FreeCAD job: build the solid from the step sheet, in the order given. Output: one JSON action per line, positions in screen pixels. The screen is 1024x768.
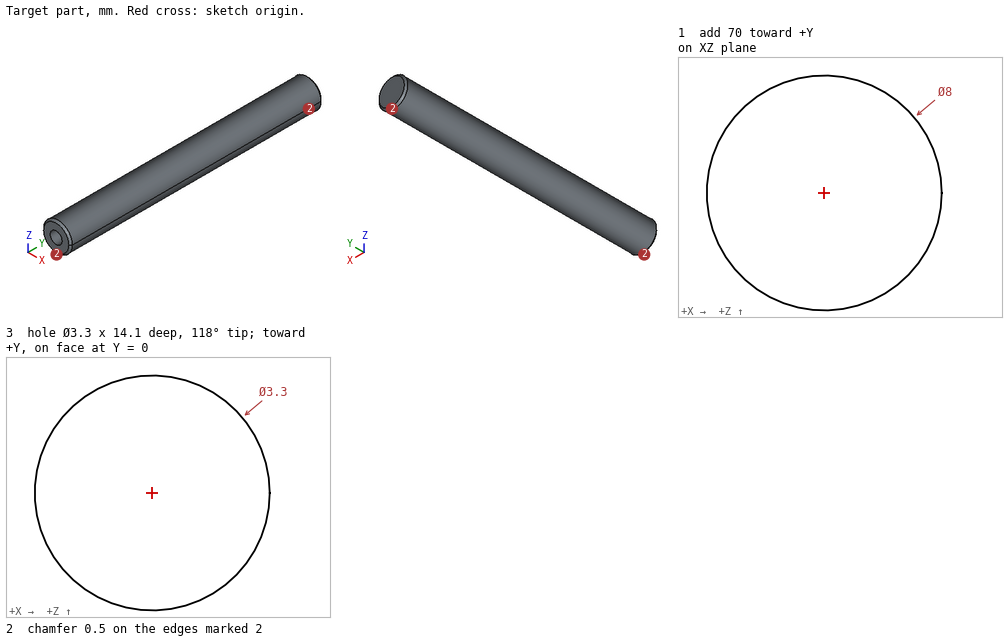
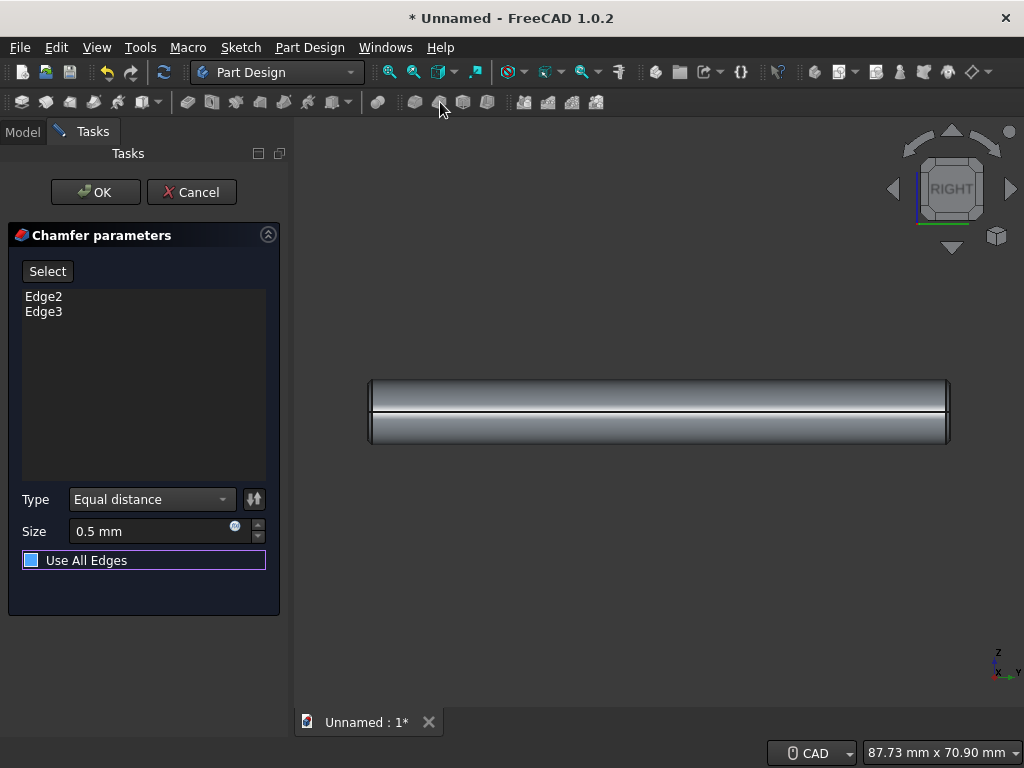
{"action": "left_click", "coordinate": [96, 192]}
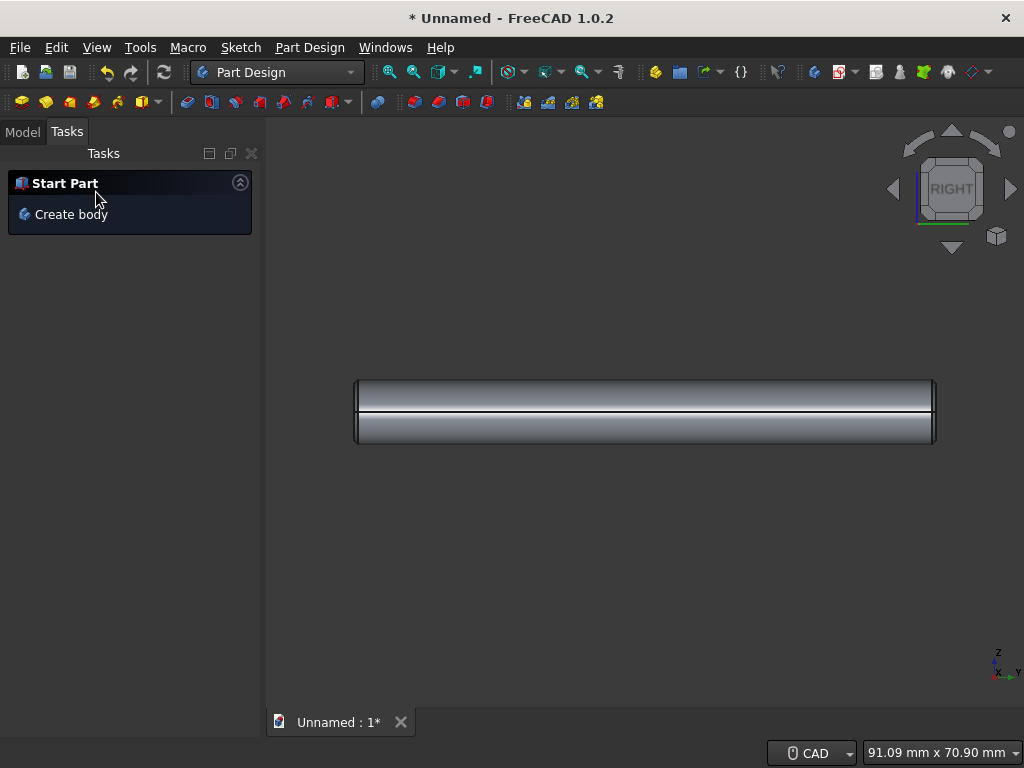
{"action": "key", "text": "0"}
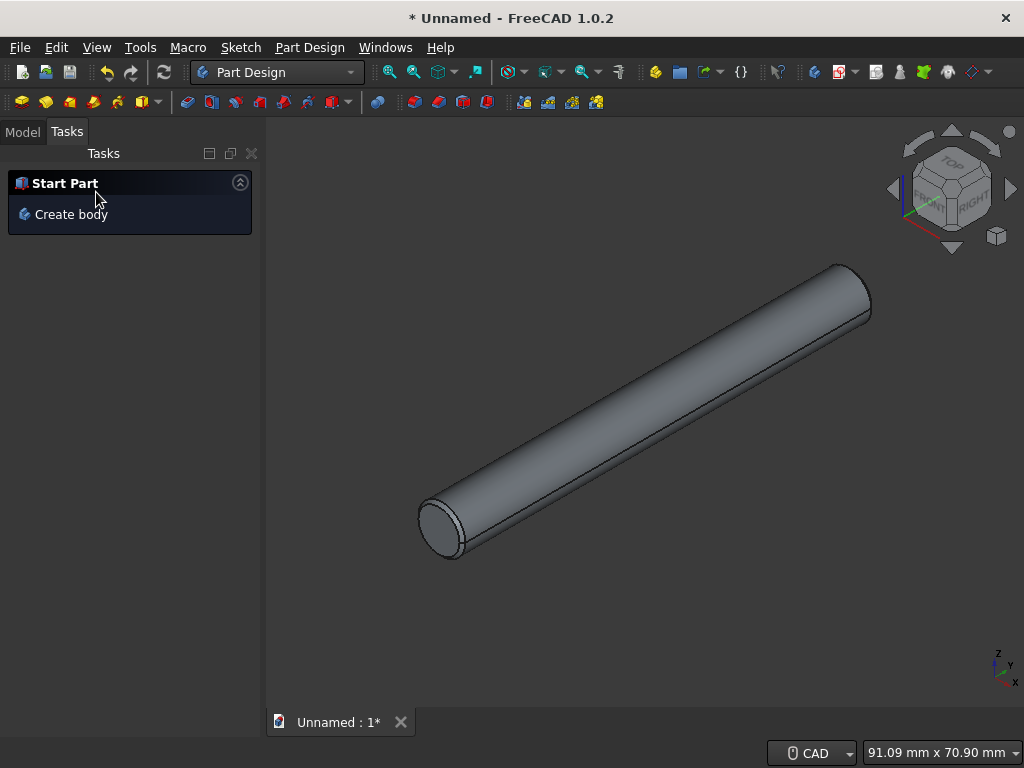
{"action": "left_click", "coordinate": [439, 530]}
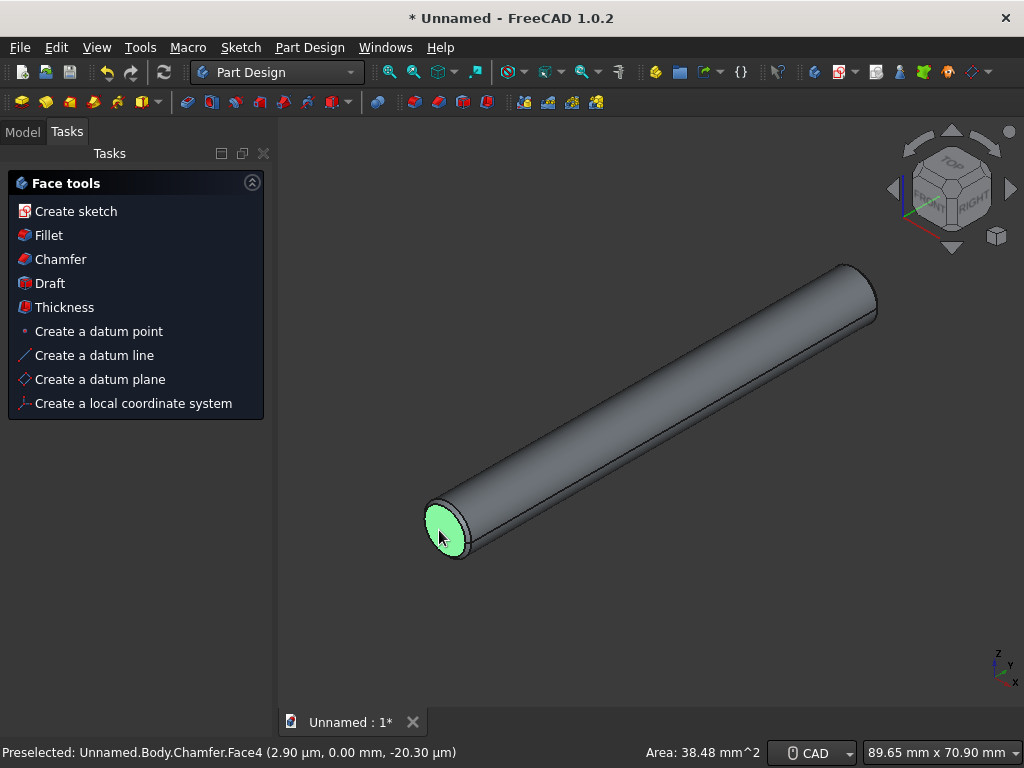
{"action": "left_click", "coordinate": [840, 72]}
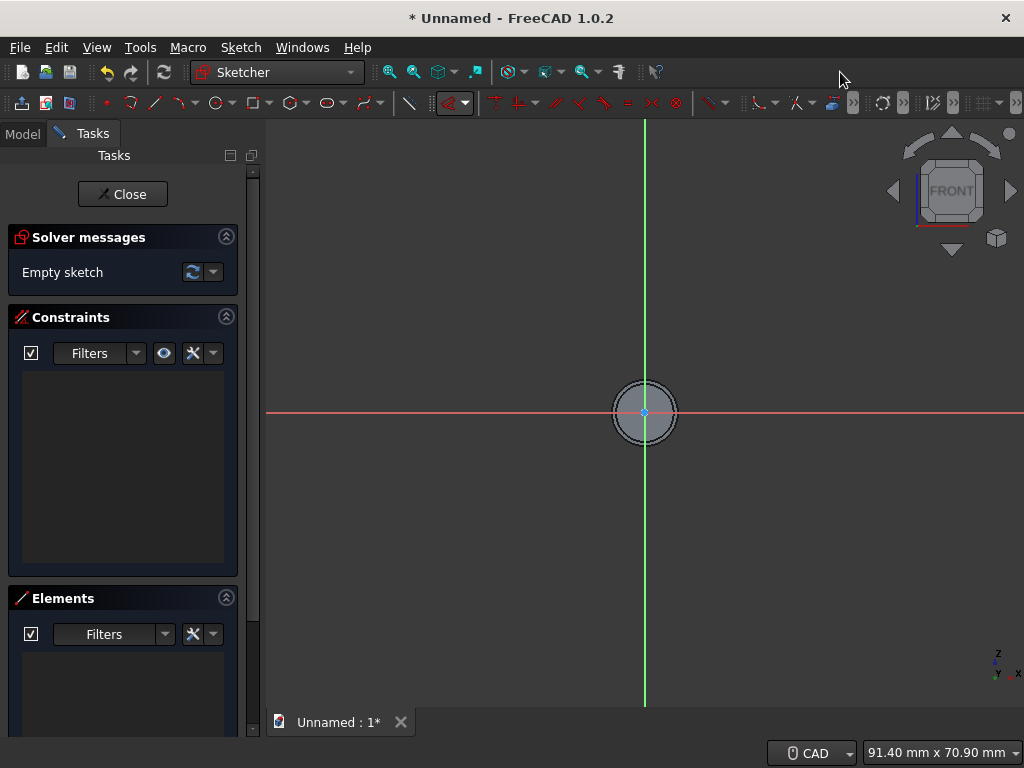
{"action": "scroll", "coordinate": [650, 413], "scroll_direction": "up", "scroll_amount": 13}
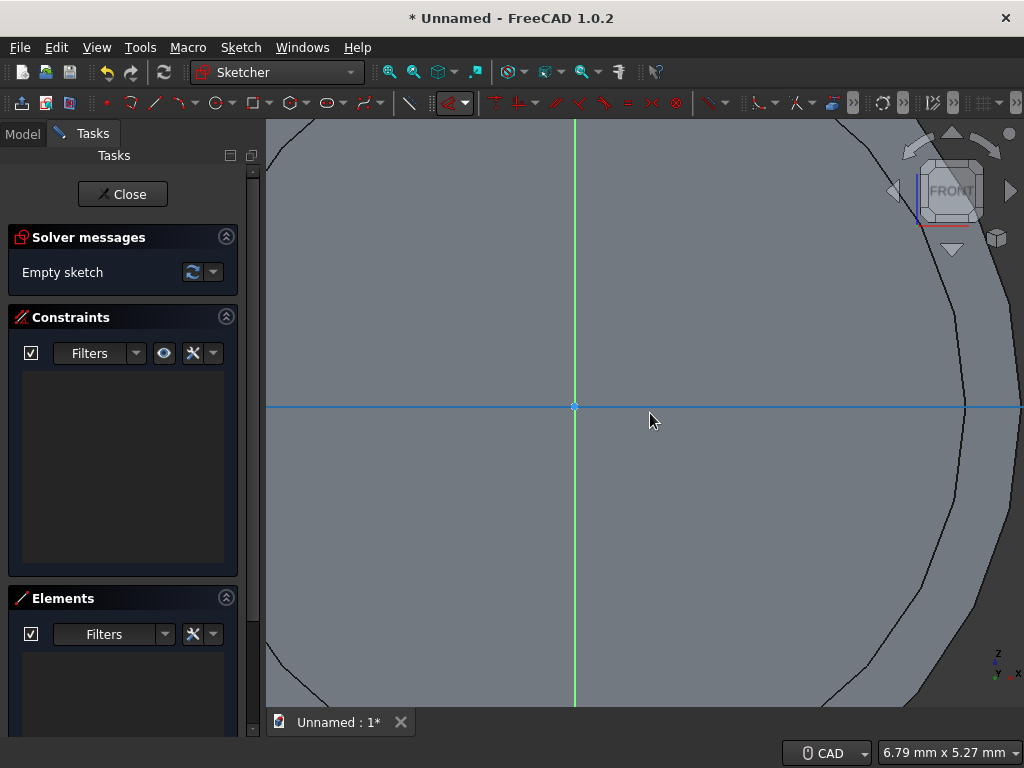
{"action": "key", "text": "g c"}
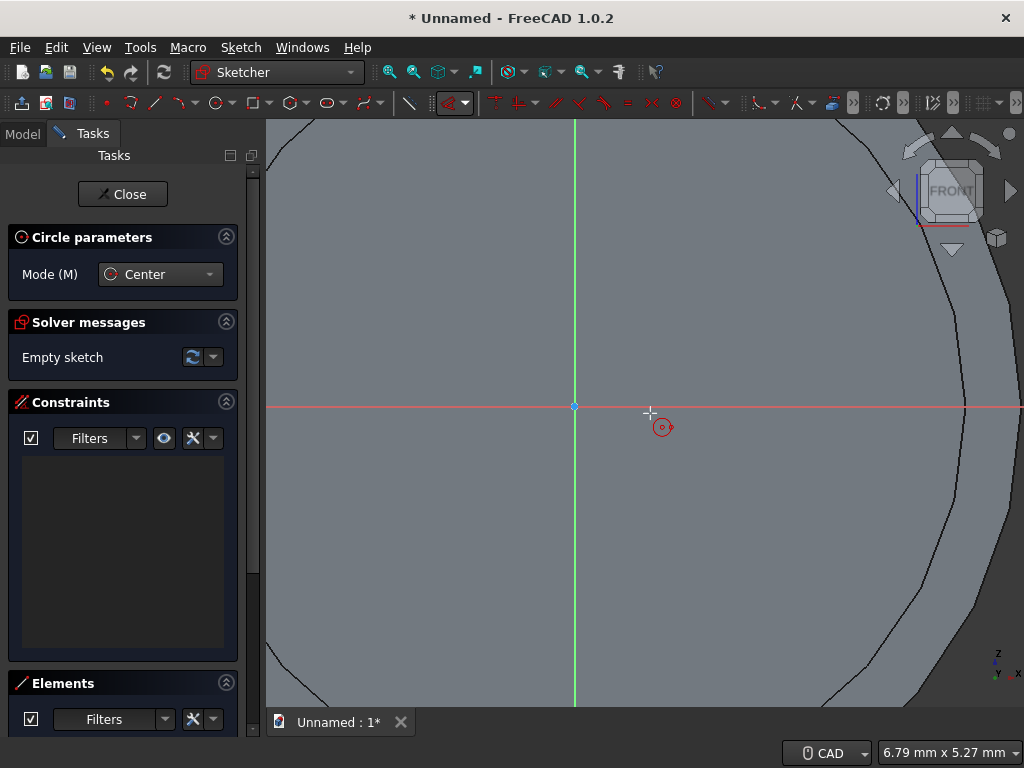
{"action": "left_click", "coordinate": [575, 407]}
{"action": "left_click", "coordinate": [705, 276]}
{"action": "key", "text": "Escape"}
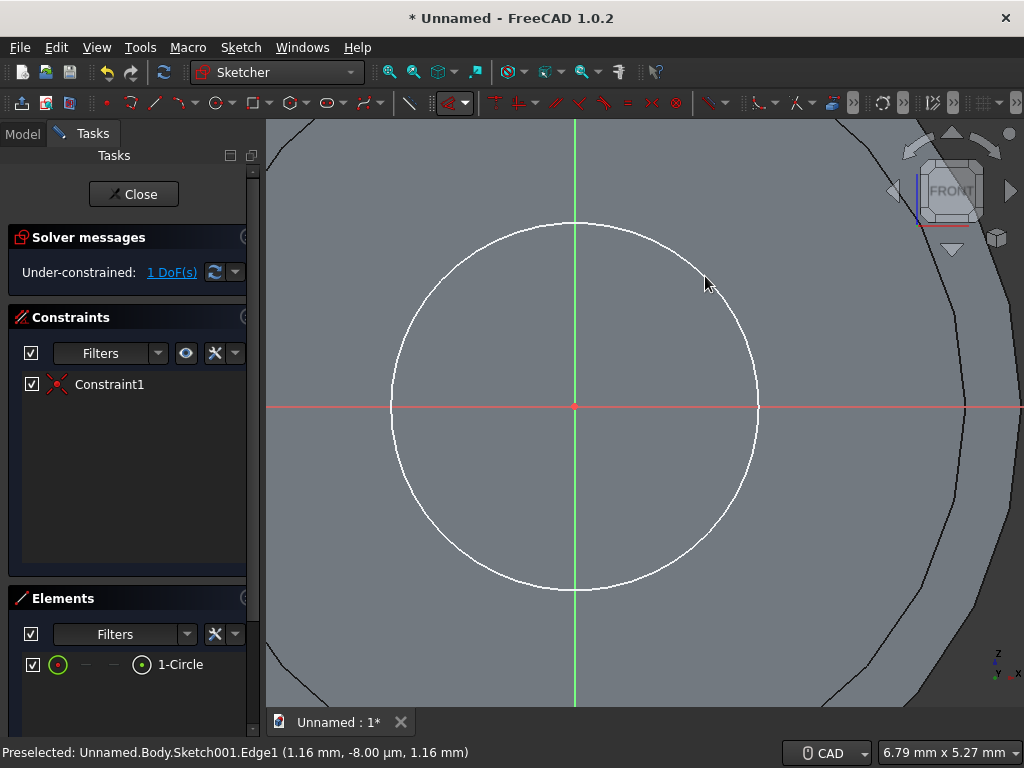
{"action": "left_click", "coordinate": [704, 276]}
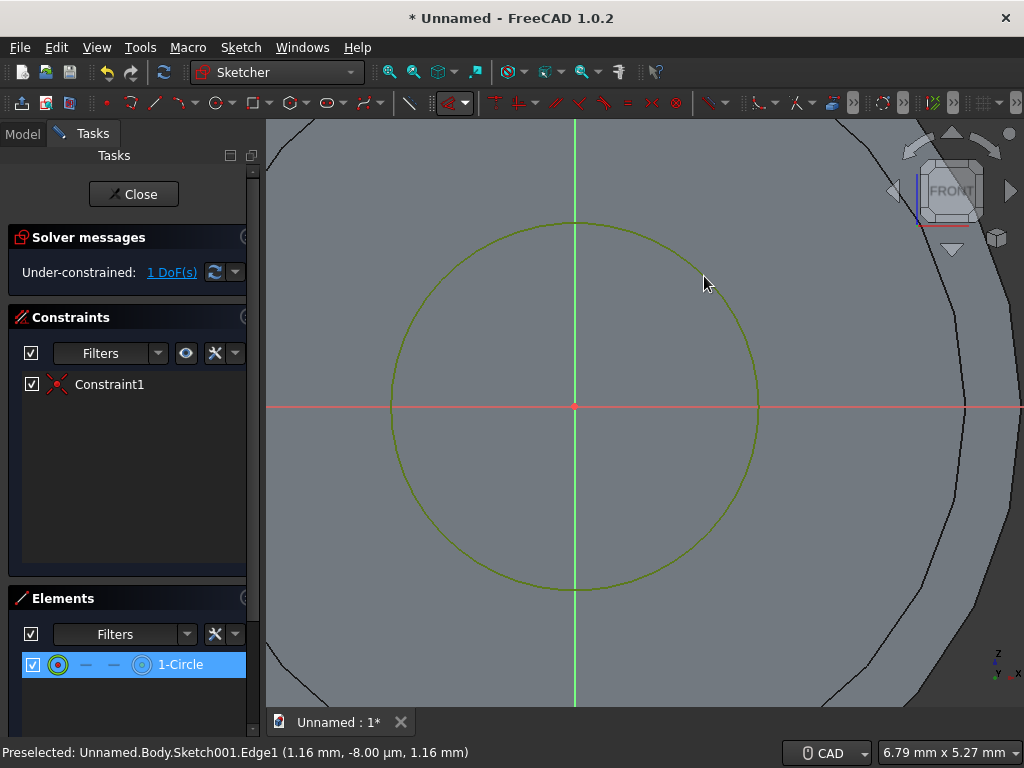
{"action": "key", "text": "k o"}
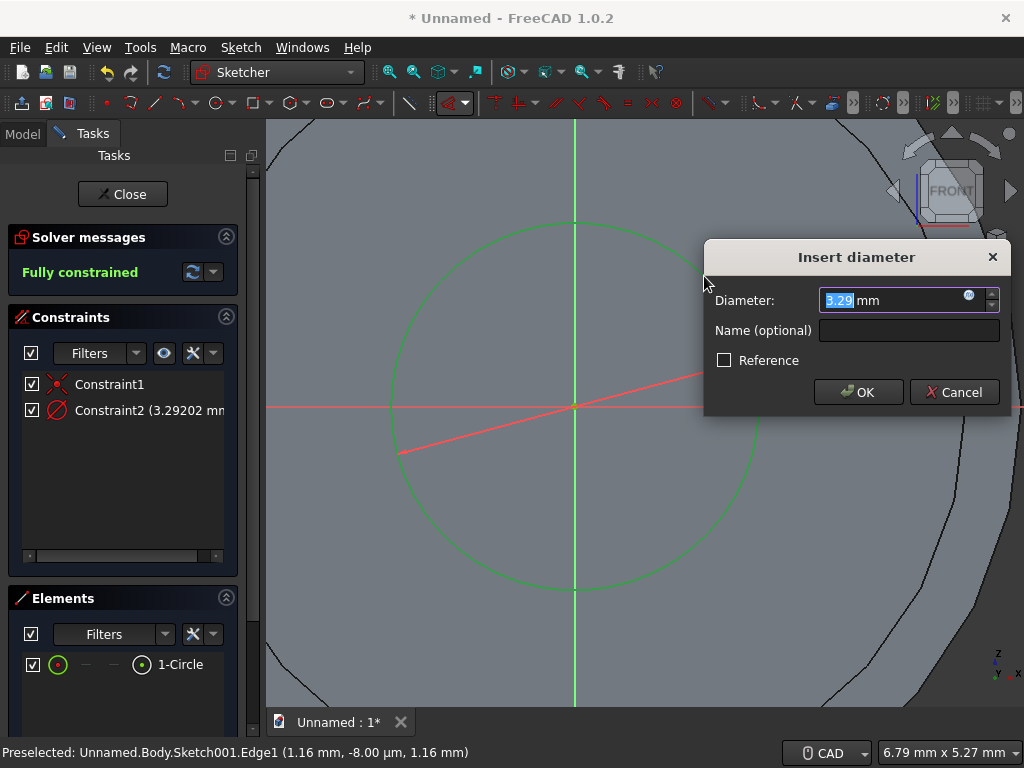
{"action": "type", "text": "3.3"}
{"action": "key", "text": "Return"}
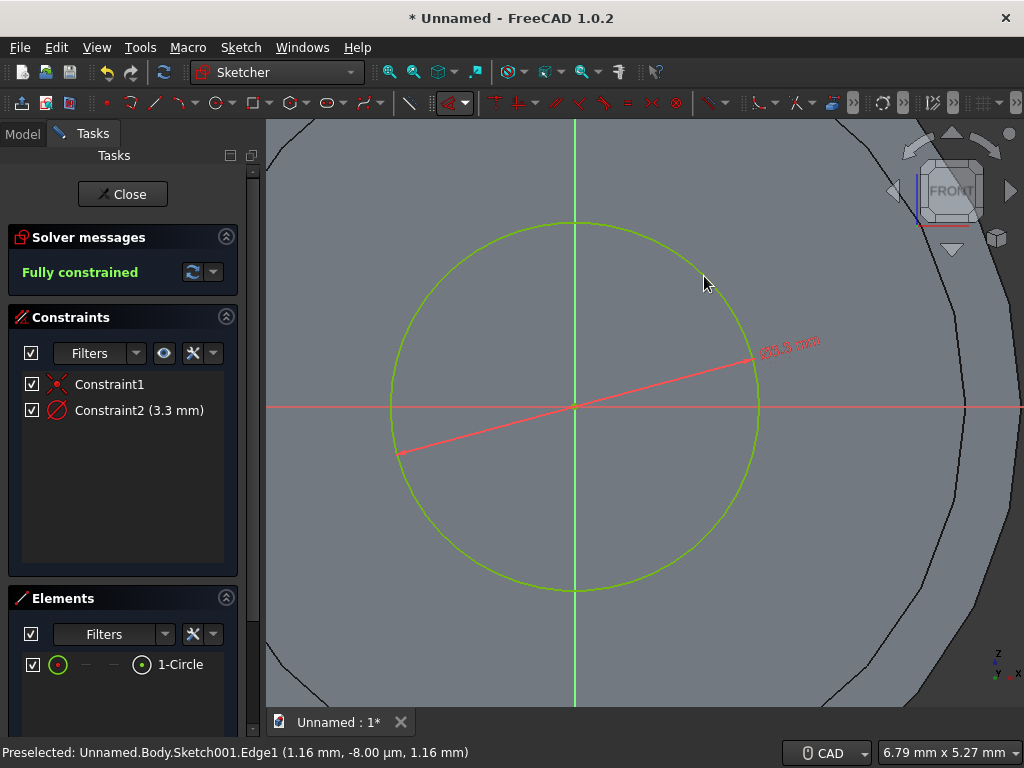
{"action": "left_click", "coordinate": [123, 194]}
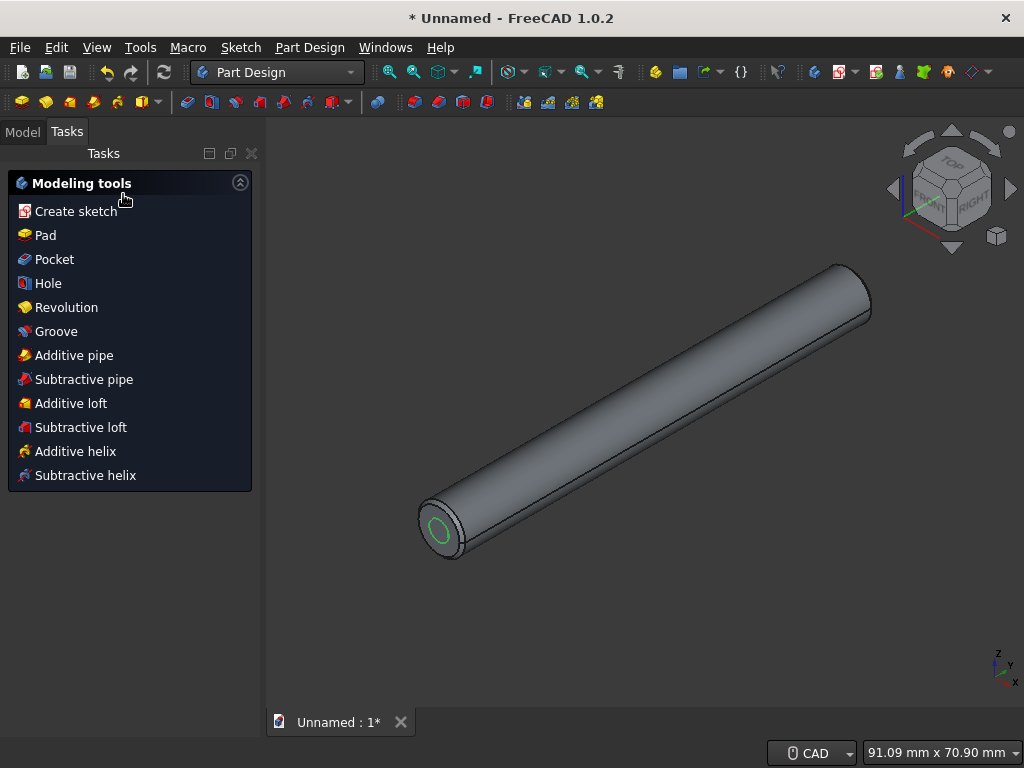
{"action": "left_click", "coordinate": [212, 102]}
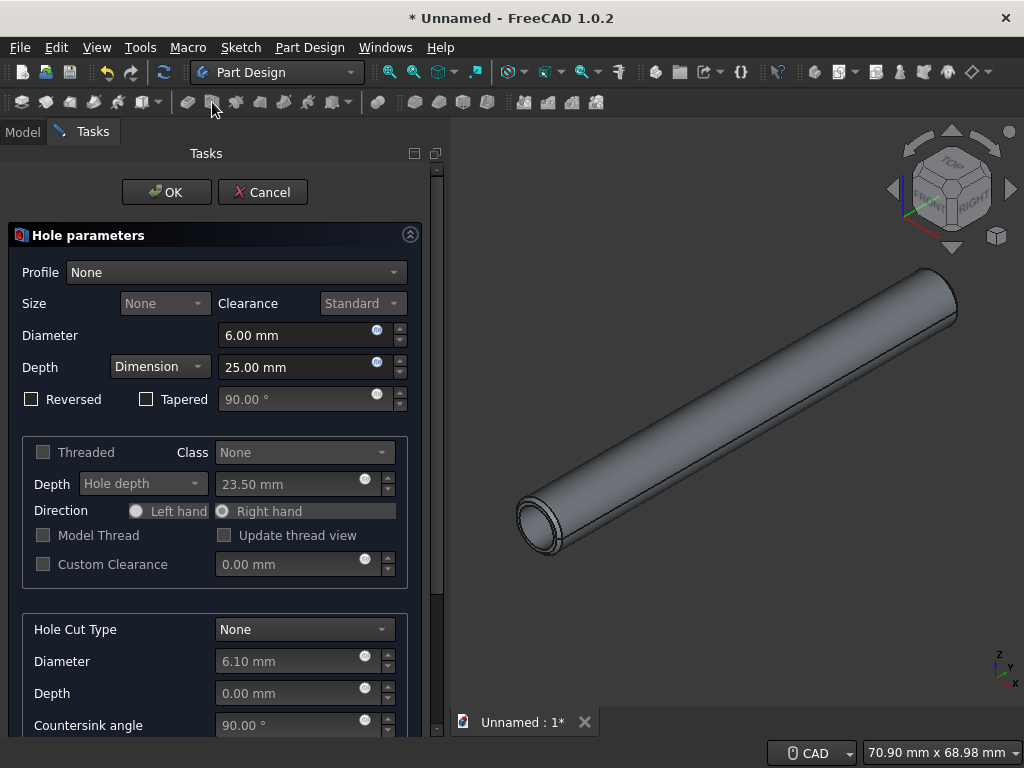
{"action": "triple_click", "coordinate": [305, 335]}